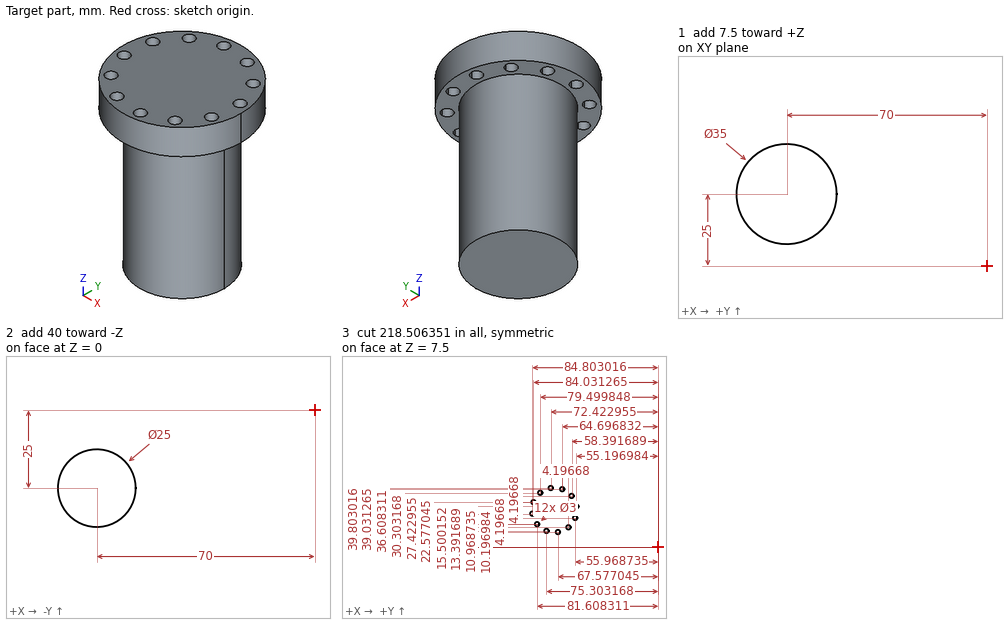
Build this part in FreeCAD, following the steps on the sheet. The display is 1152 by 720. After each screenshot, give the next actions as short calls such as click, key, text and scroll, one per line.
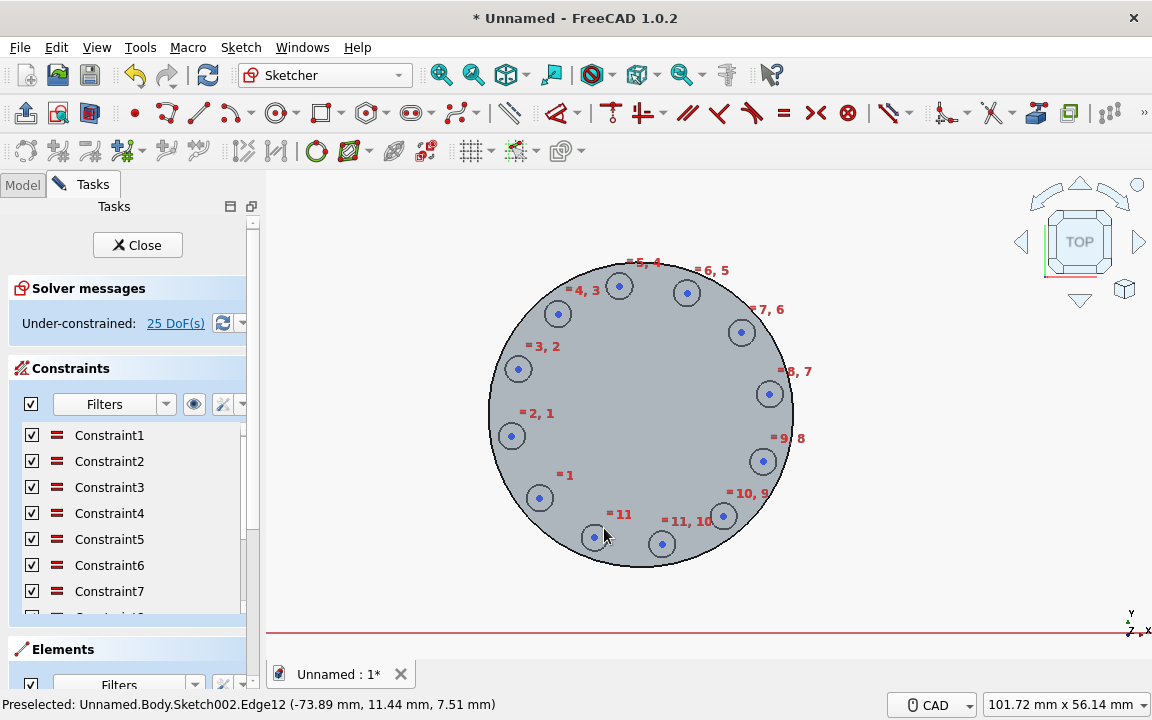
click(556, 114)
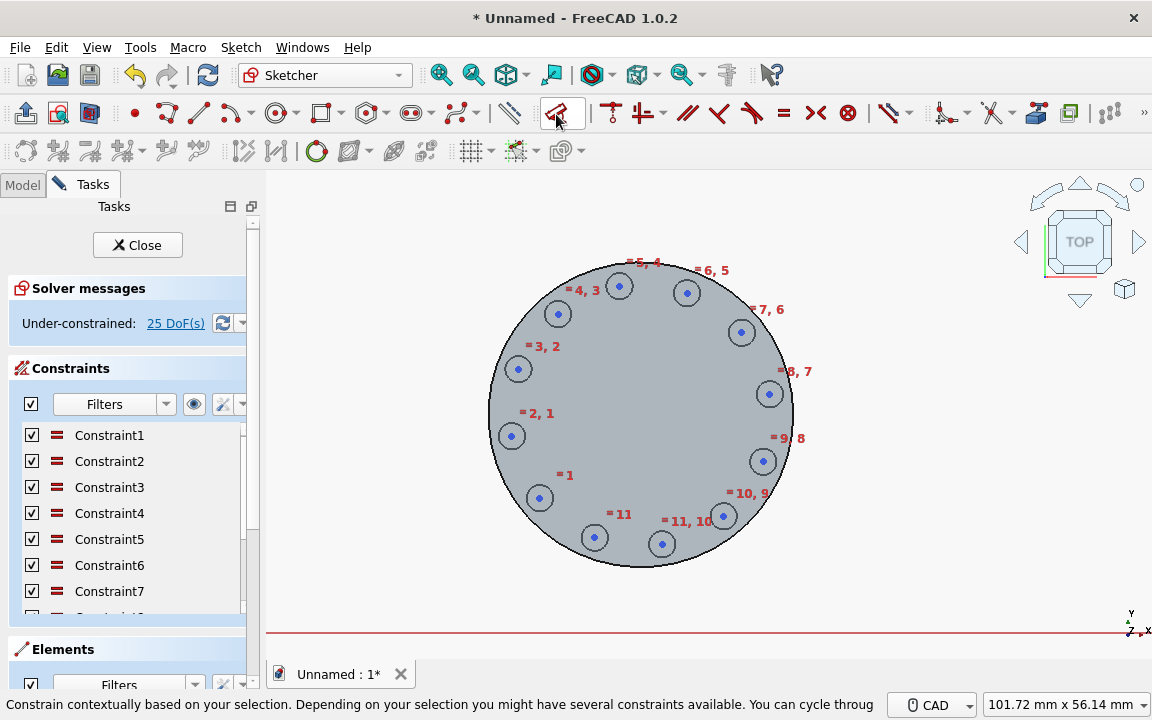
scroll(549, 489, up, 3)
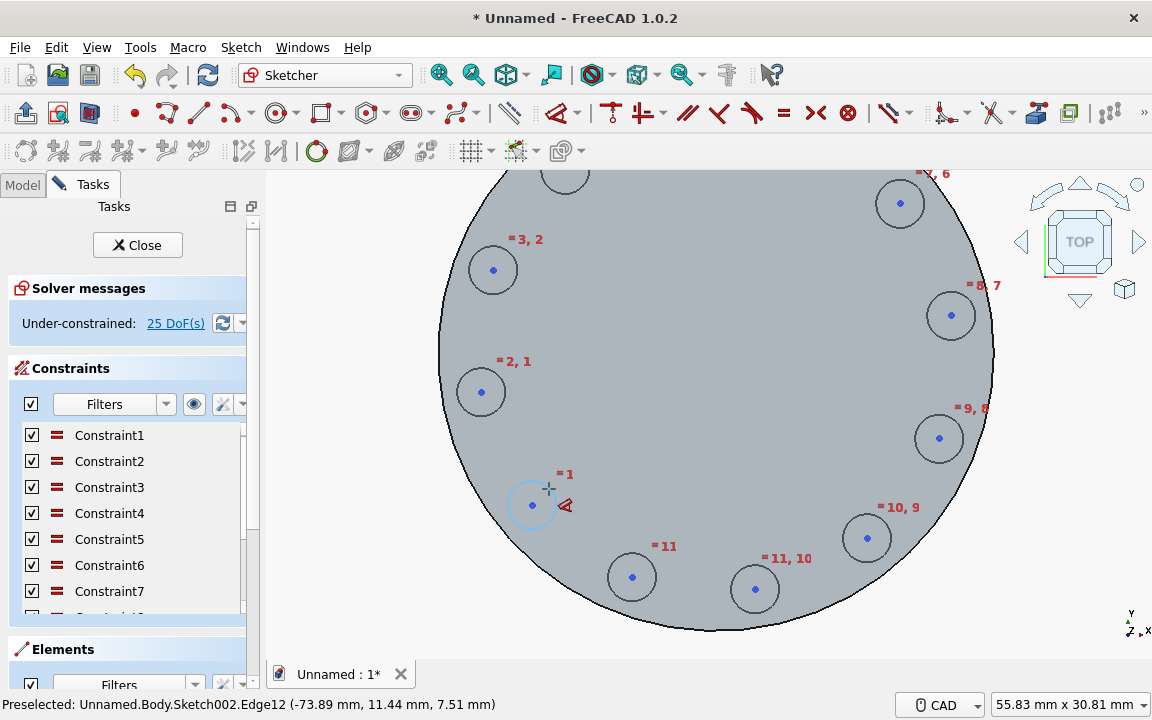
click(549, 488)
click(571, 465)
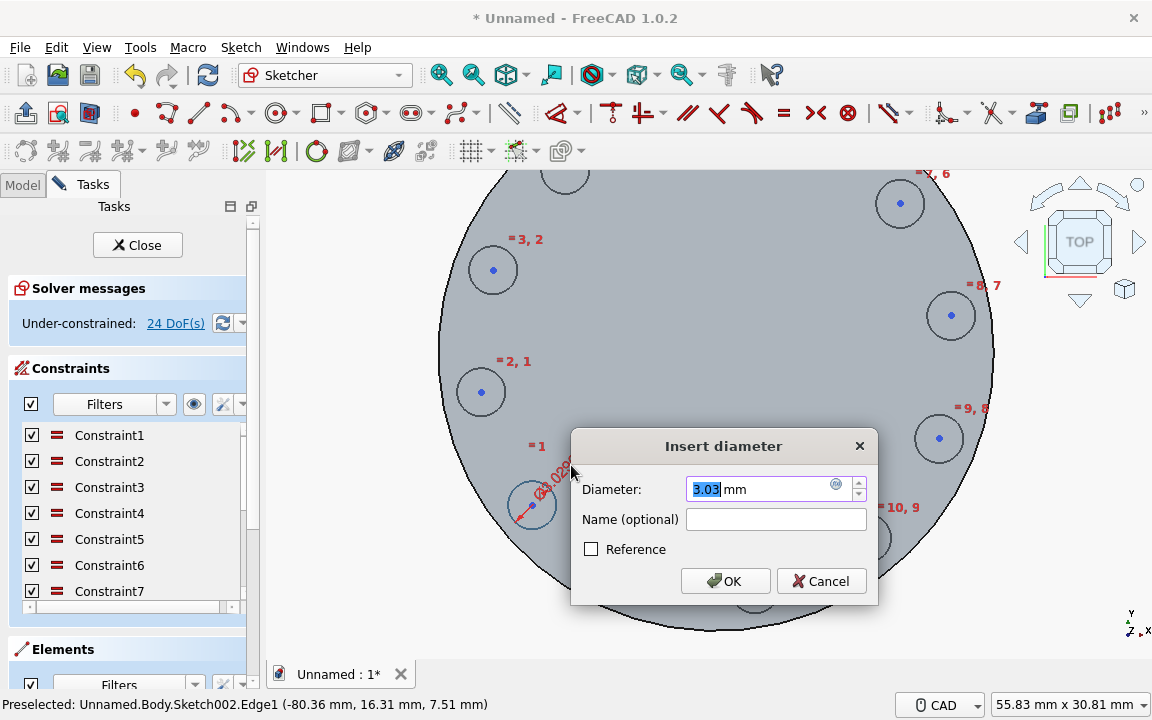
text(3)
key(Return)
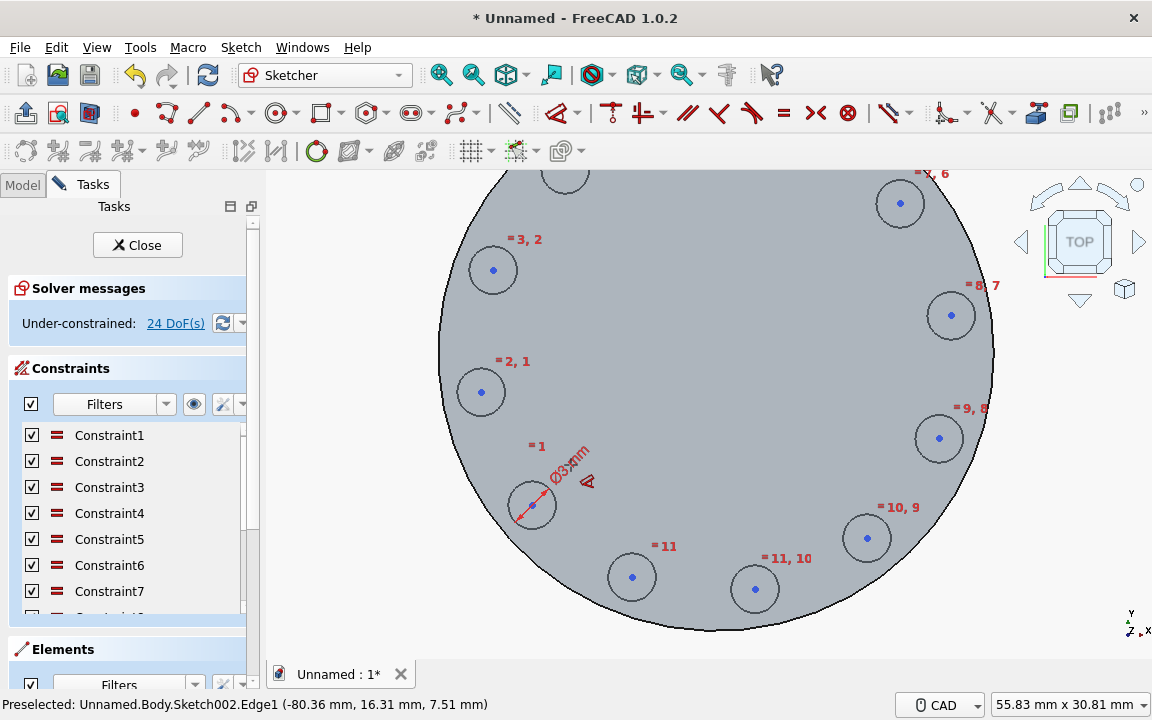
click(493, 270)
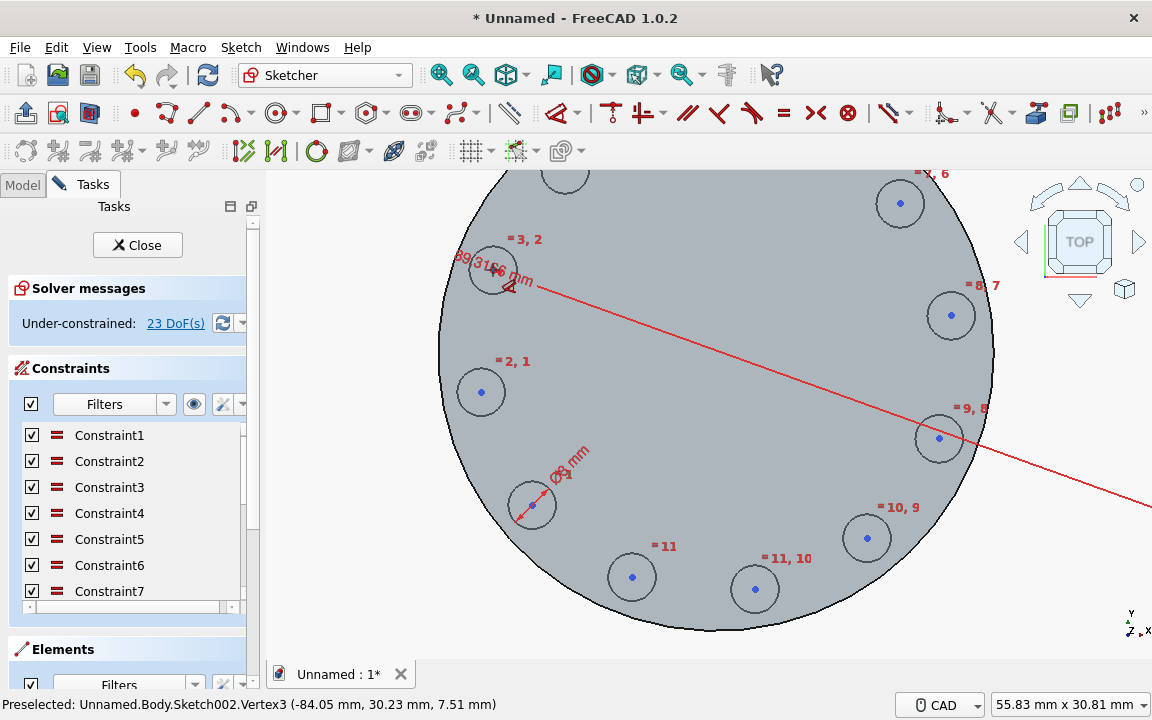
click(900, 204)
click(459, 237)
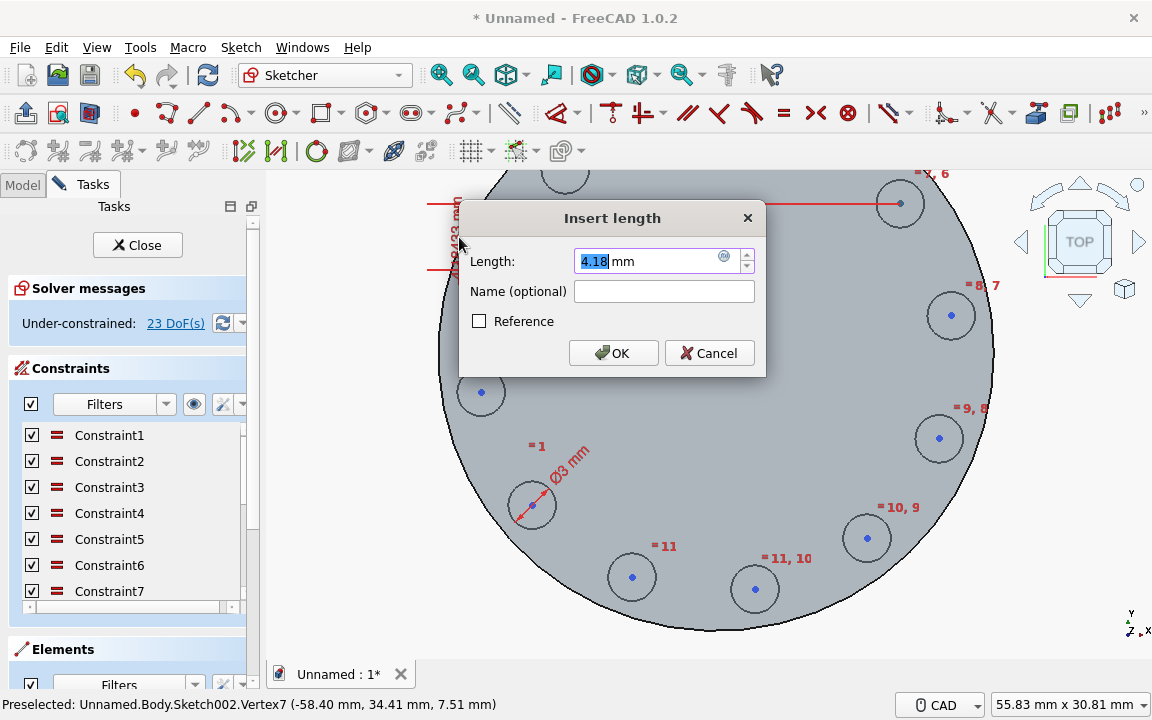
text(4.19668)
key(Return)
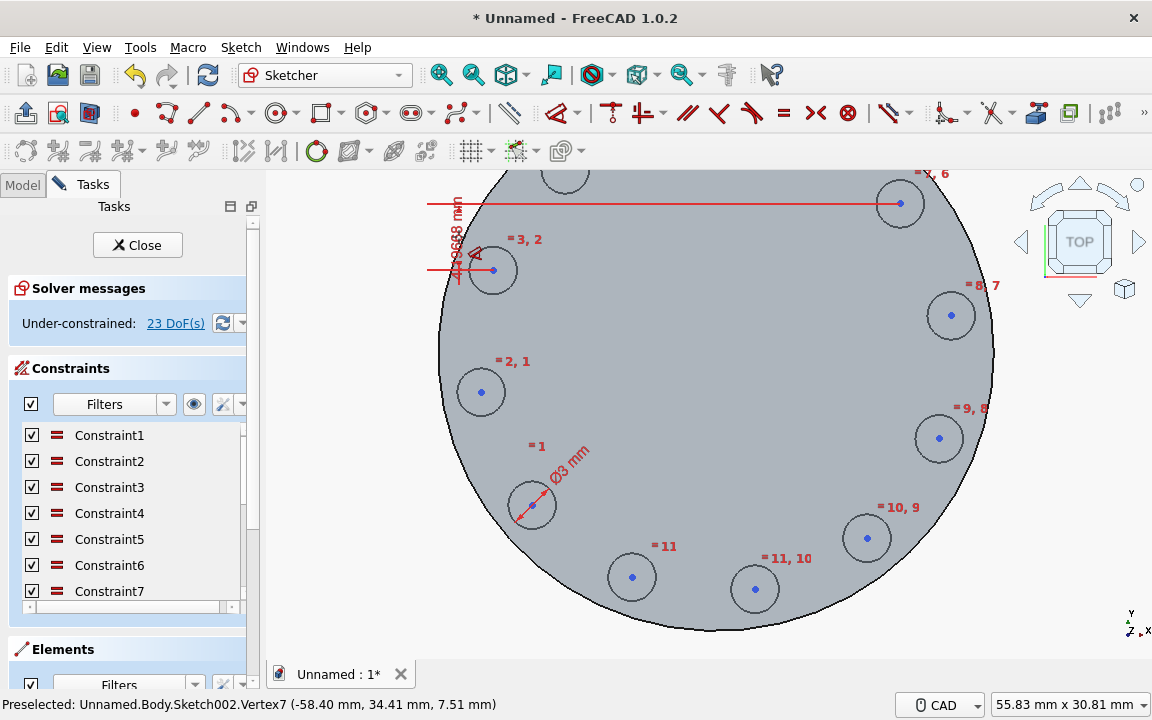
click(532, 505)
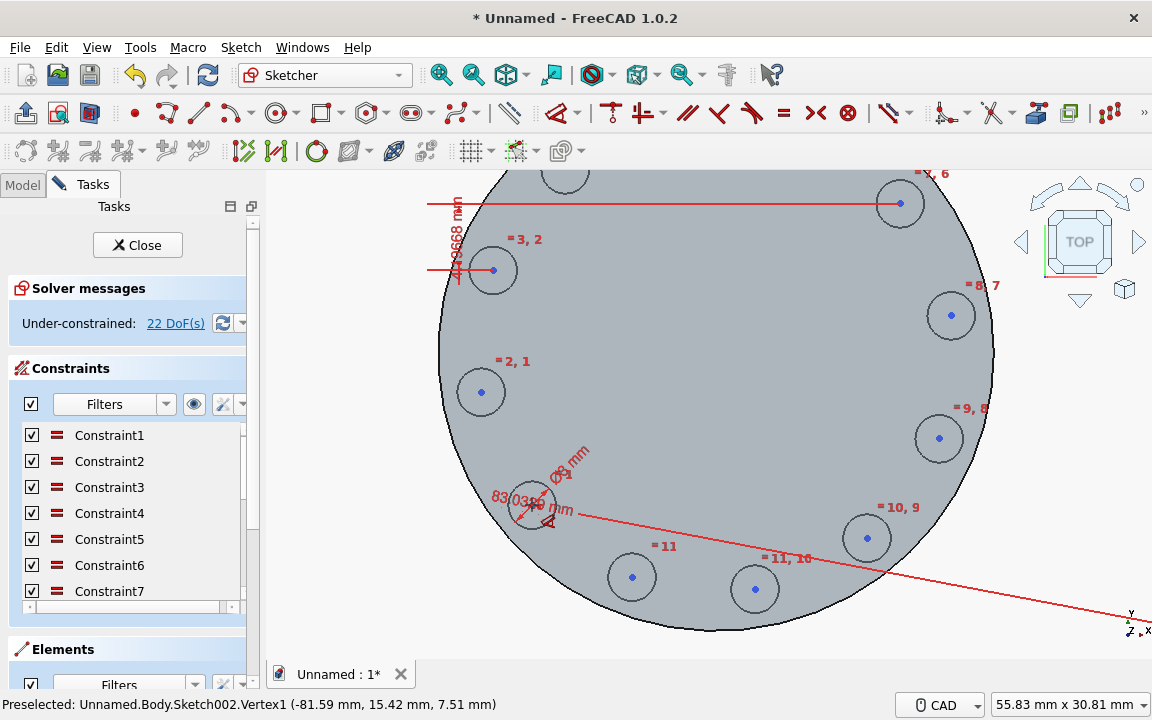
click(939, 439)
click(973, 472)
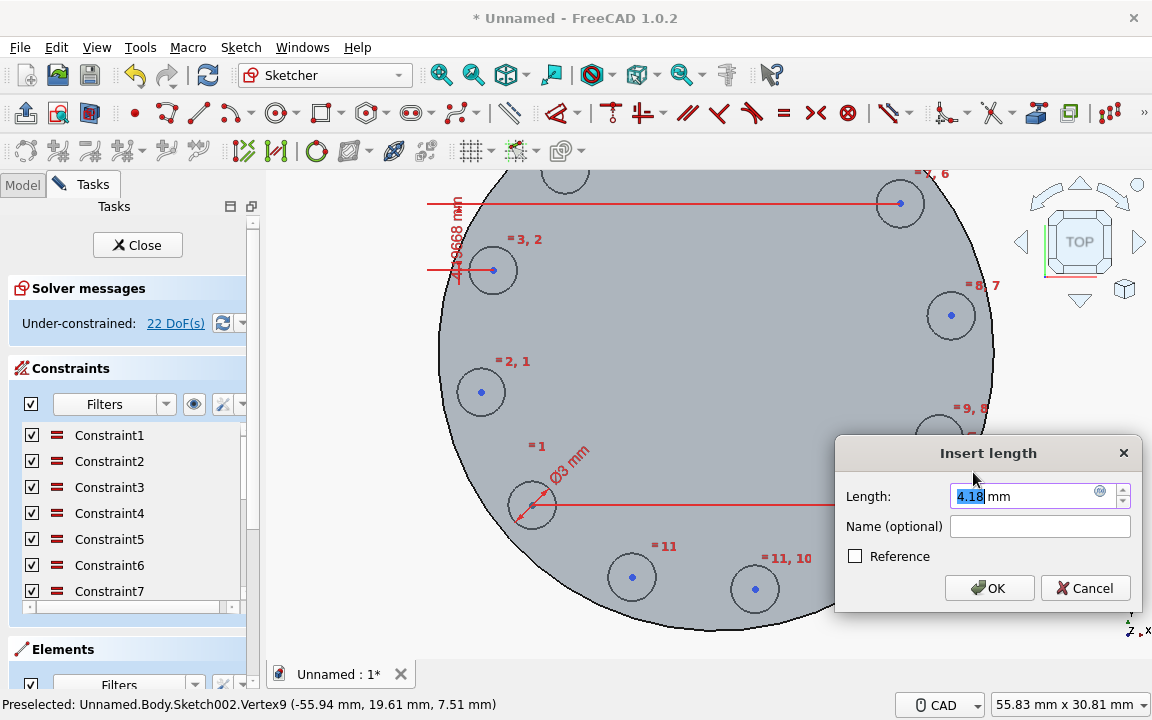
text(4.19668)
key(Return)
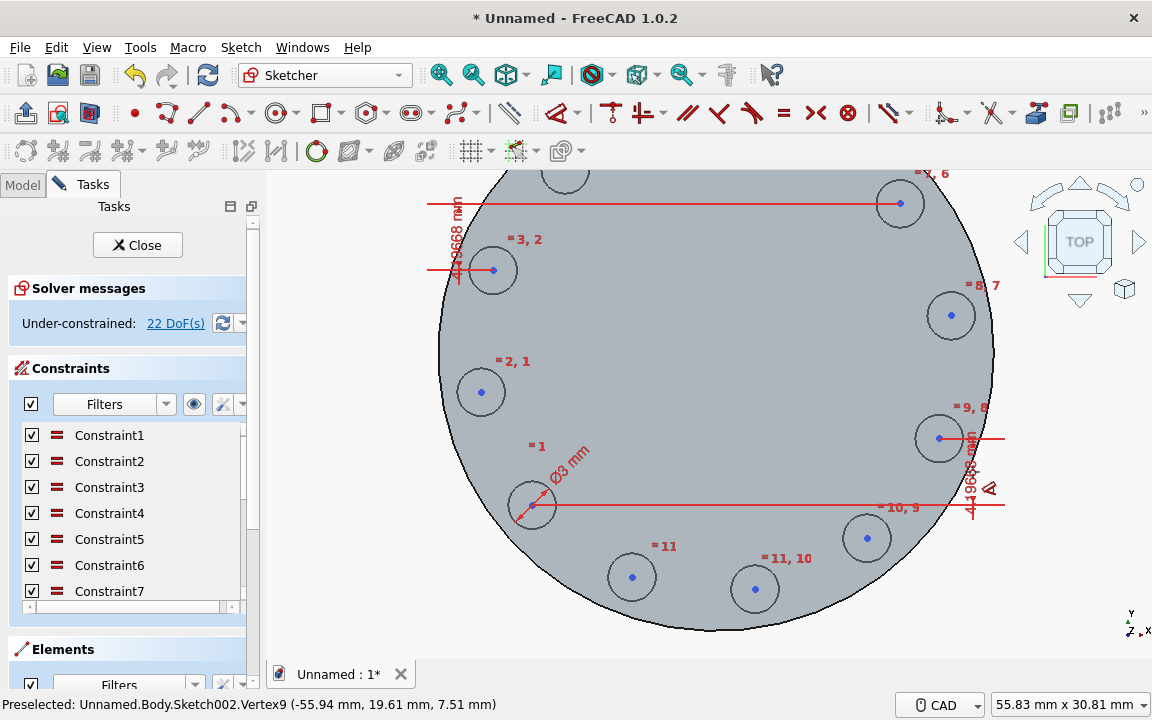
scroll(549, 489, down, 3)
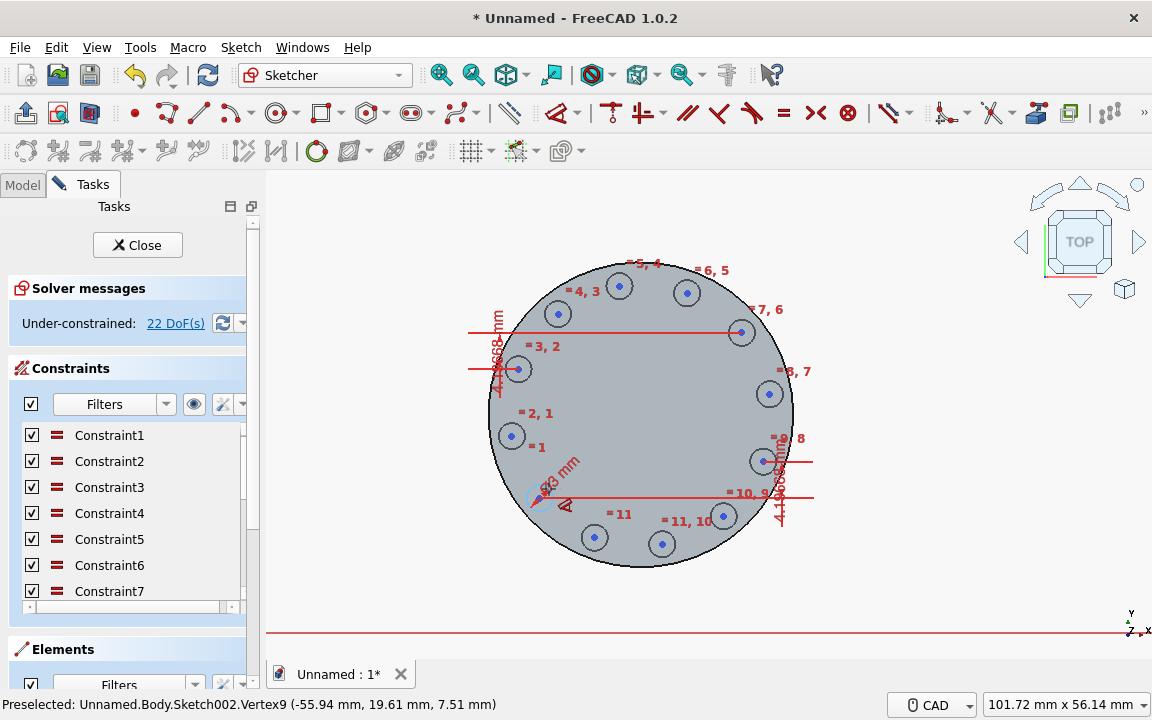
click(687, 293)